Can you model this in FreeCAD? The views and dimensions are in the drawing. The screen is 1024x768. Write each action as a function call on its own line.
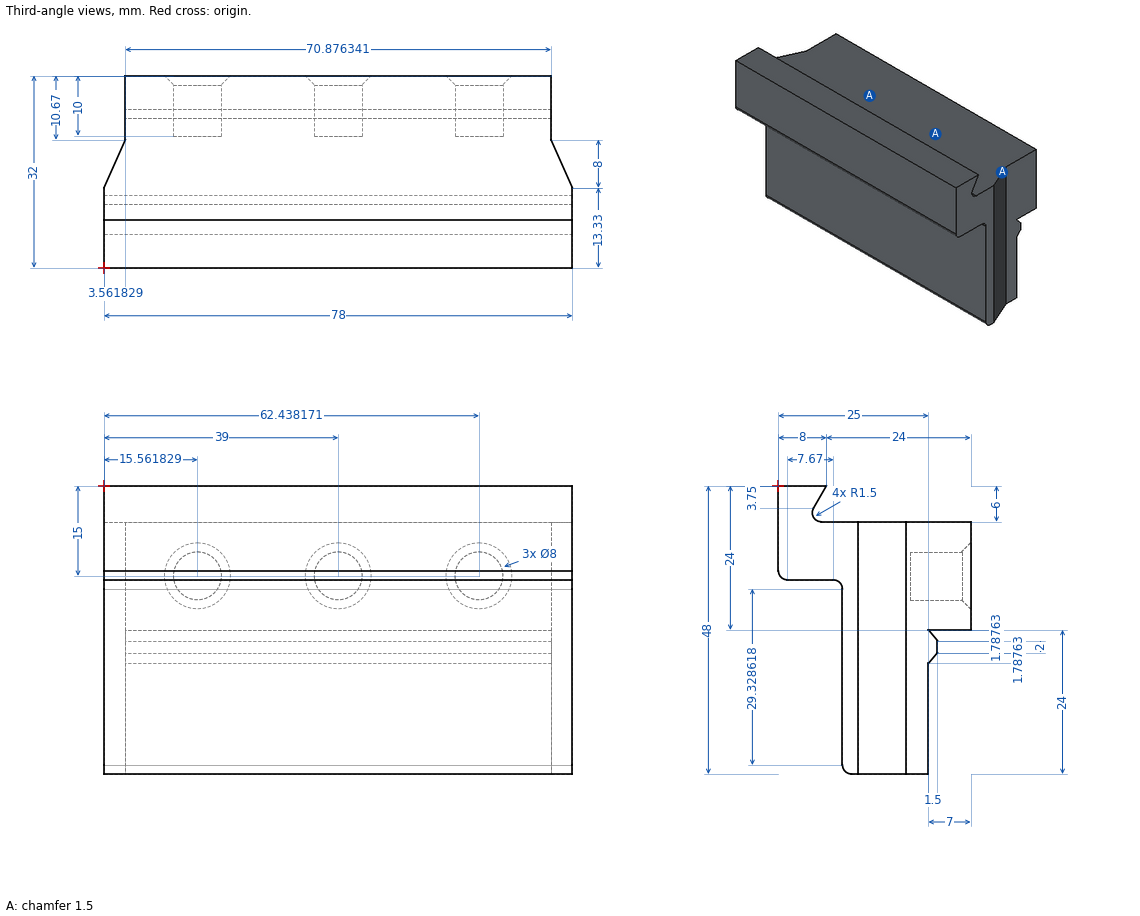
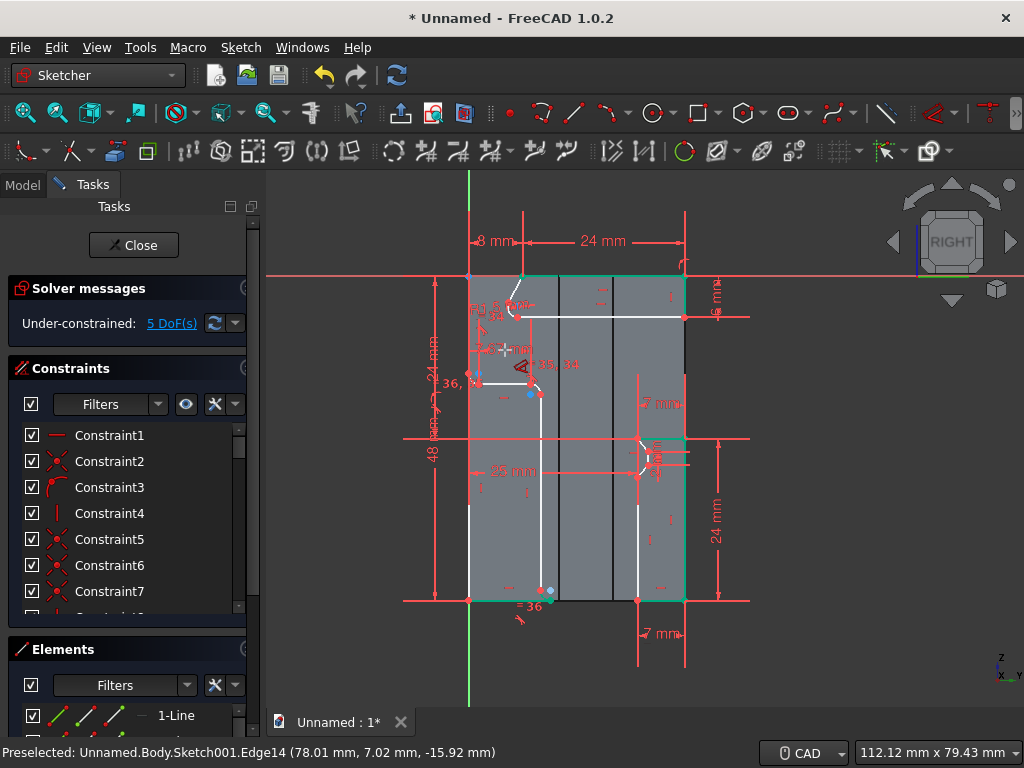
scroll(644, 447, up, 7)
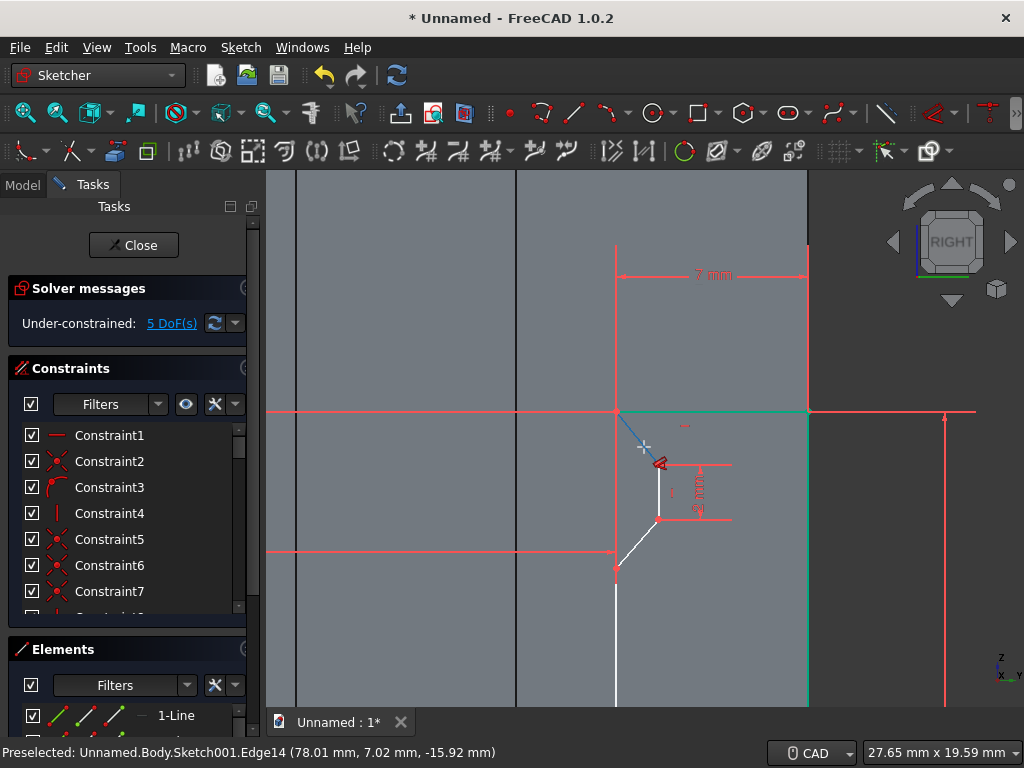
click(642, 444)
click(628, 499)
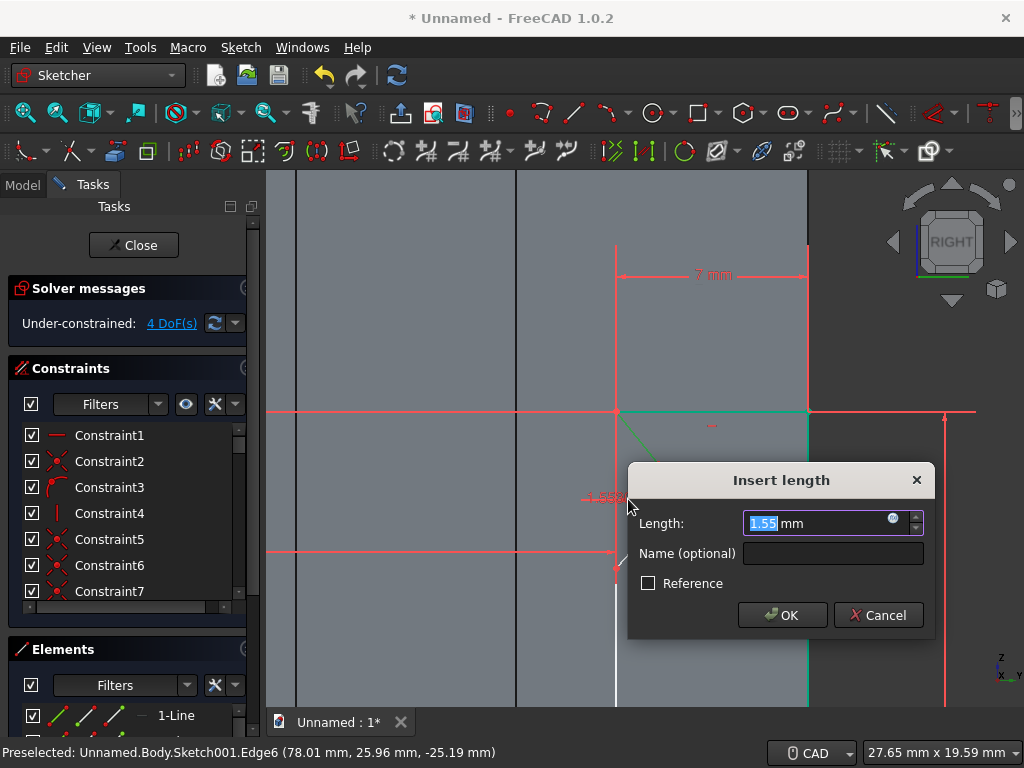
text(1.5)
key(Return)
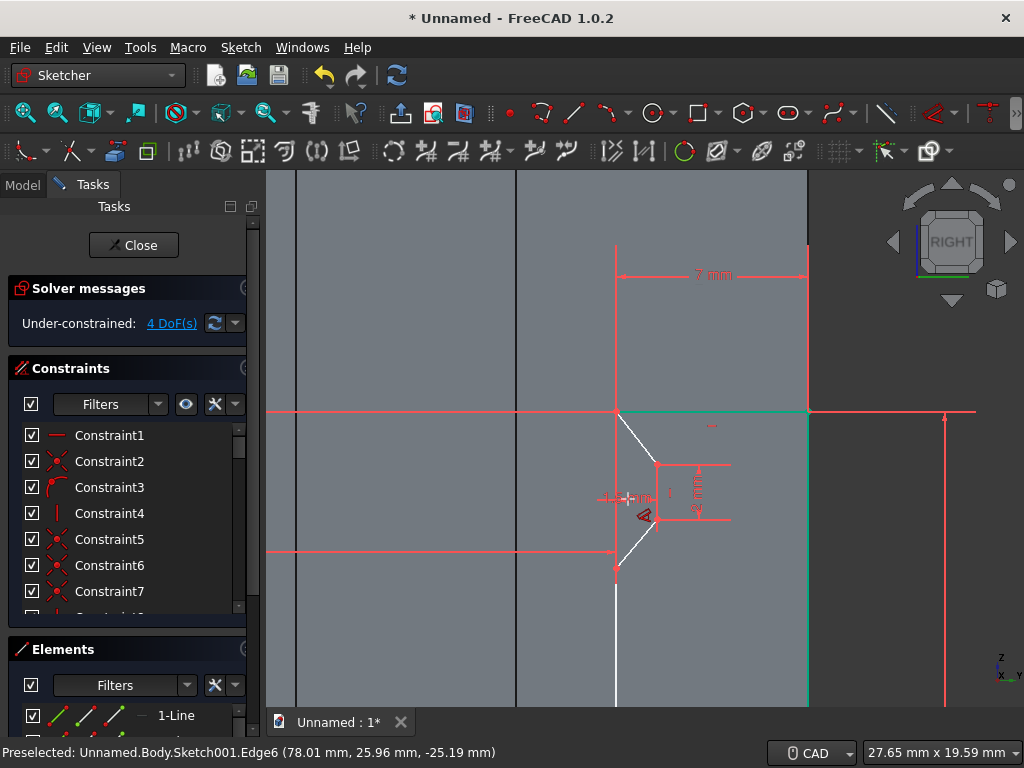
scroll(644, 447, down, 7)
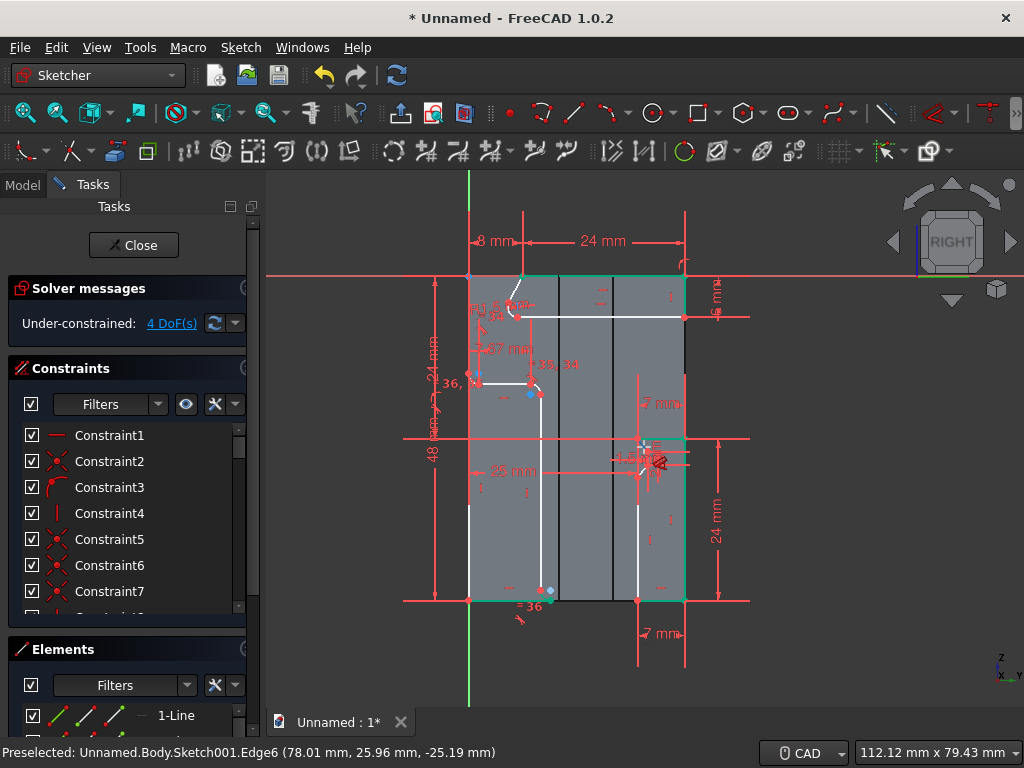
scroll(509, 302, up, 3)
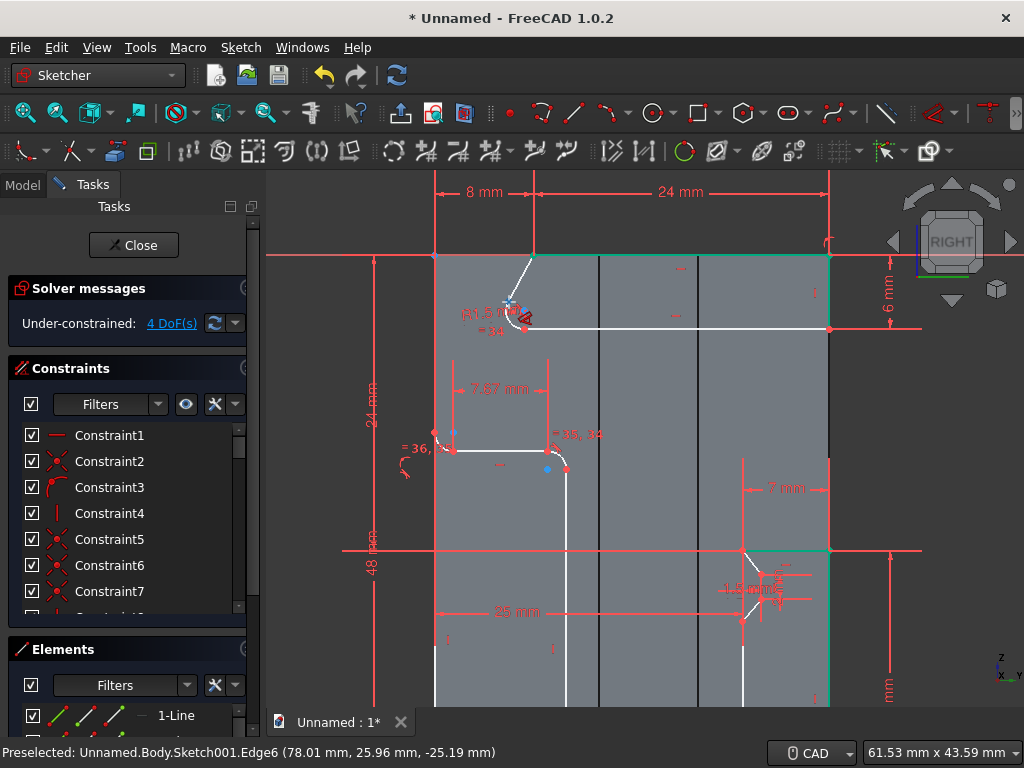
click(508, 302)
click(401, 279)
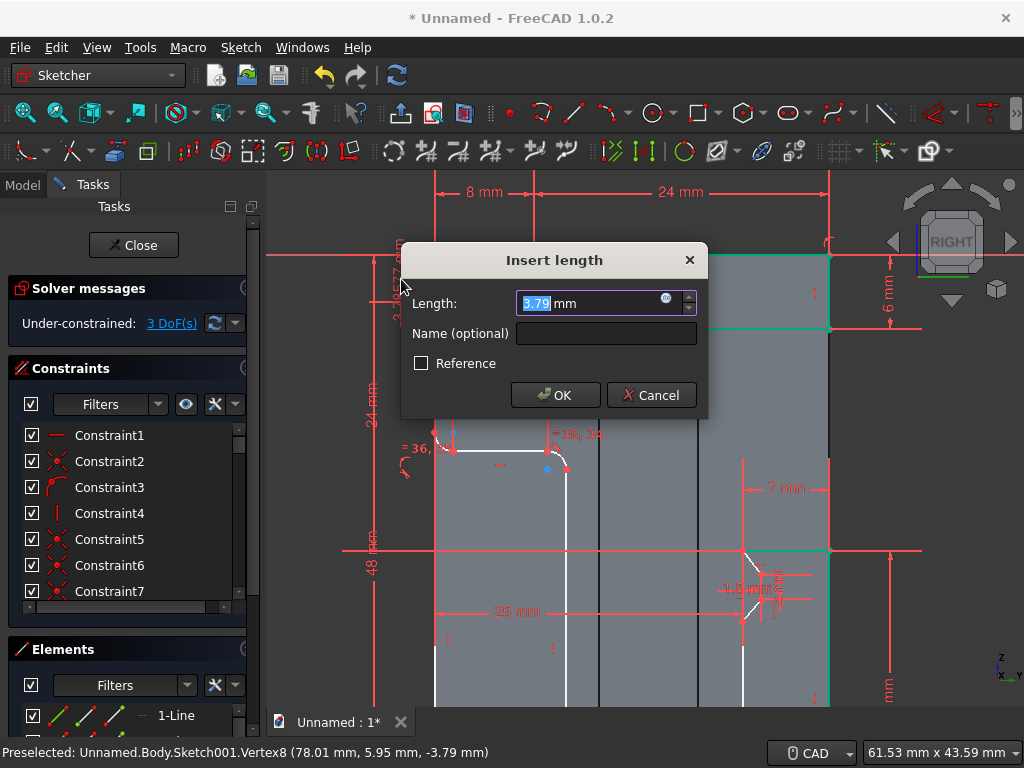
text(3.75)
key(Return)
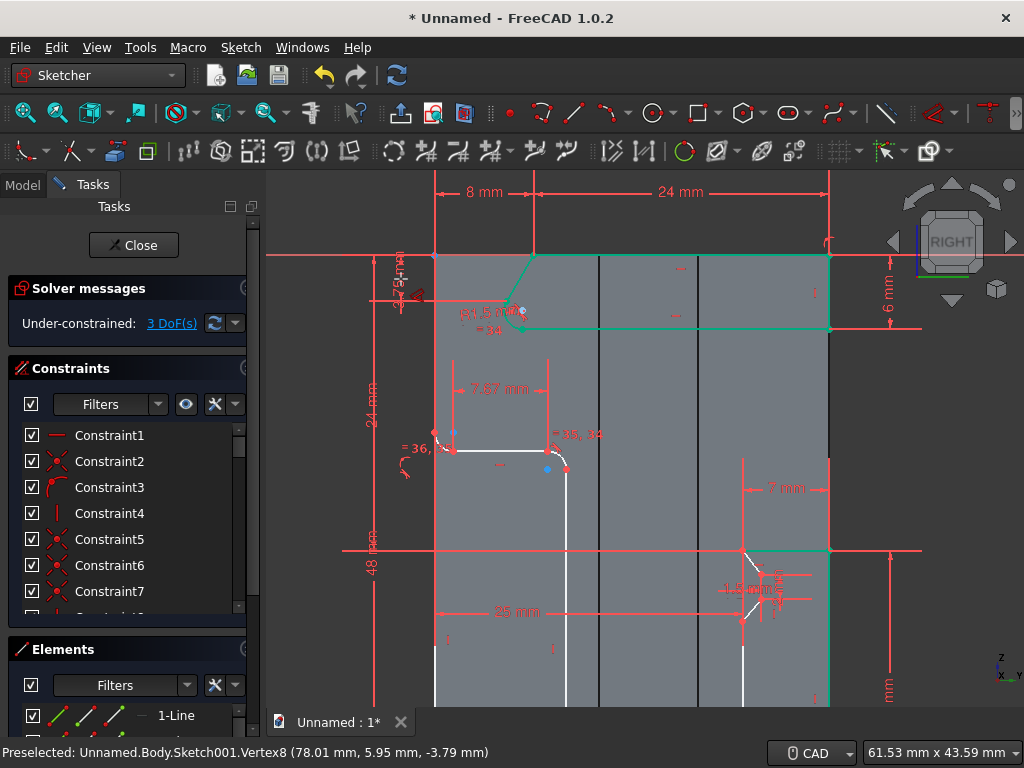
scroll(756, 568, up, 3)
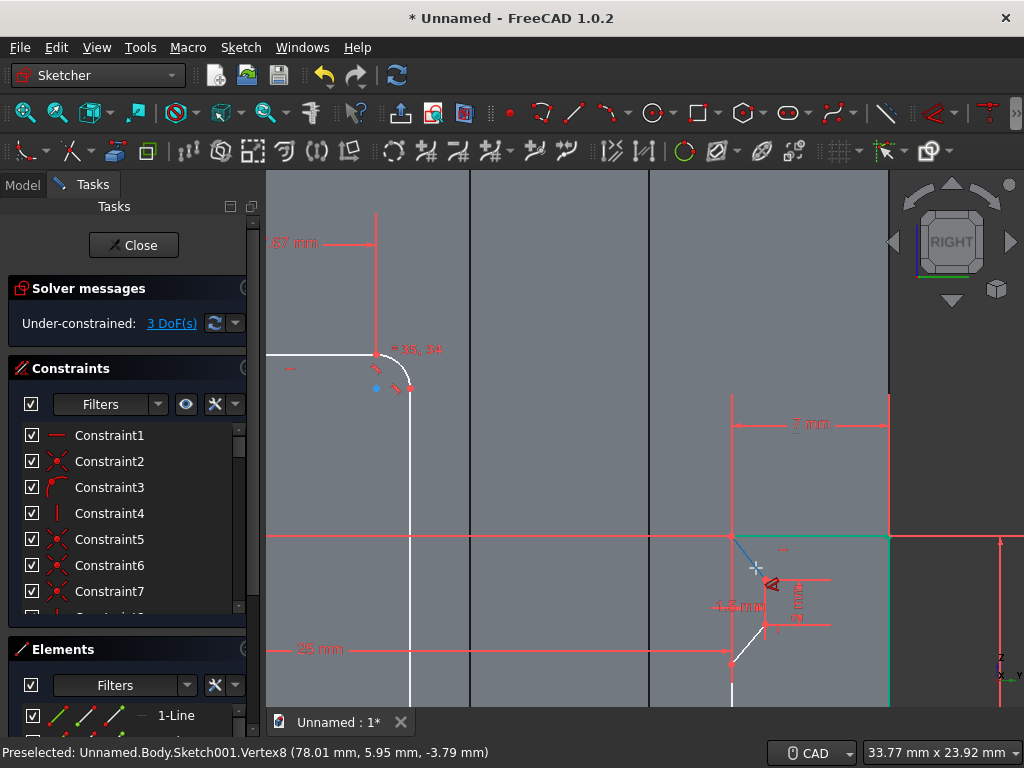
click(755, 567)
click(799, 558)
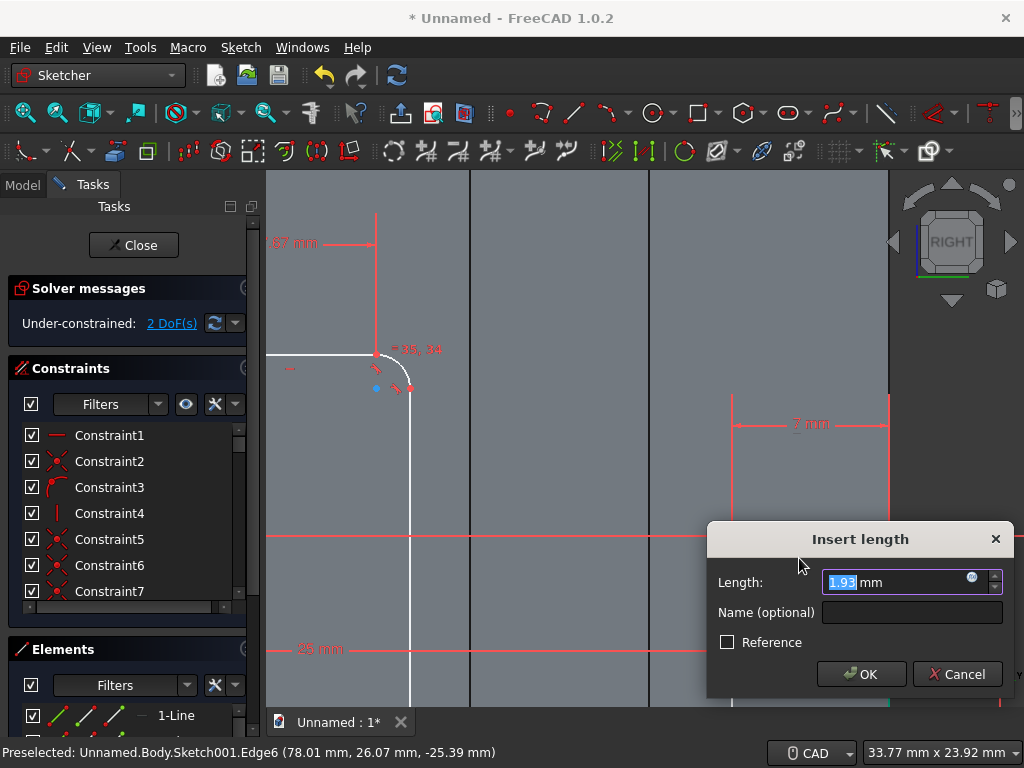
text(1.78763)
key(Return)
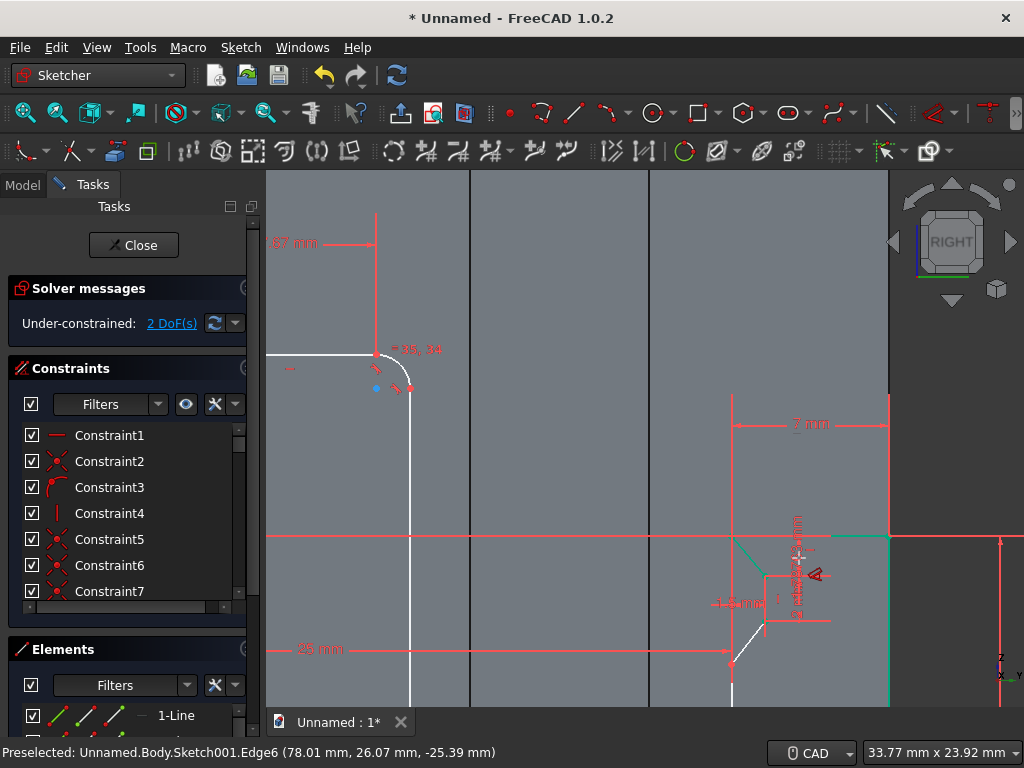
click(755, 634)
click(799, 643)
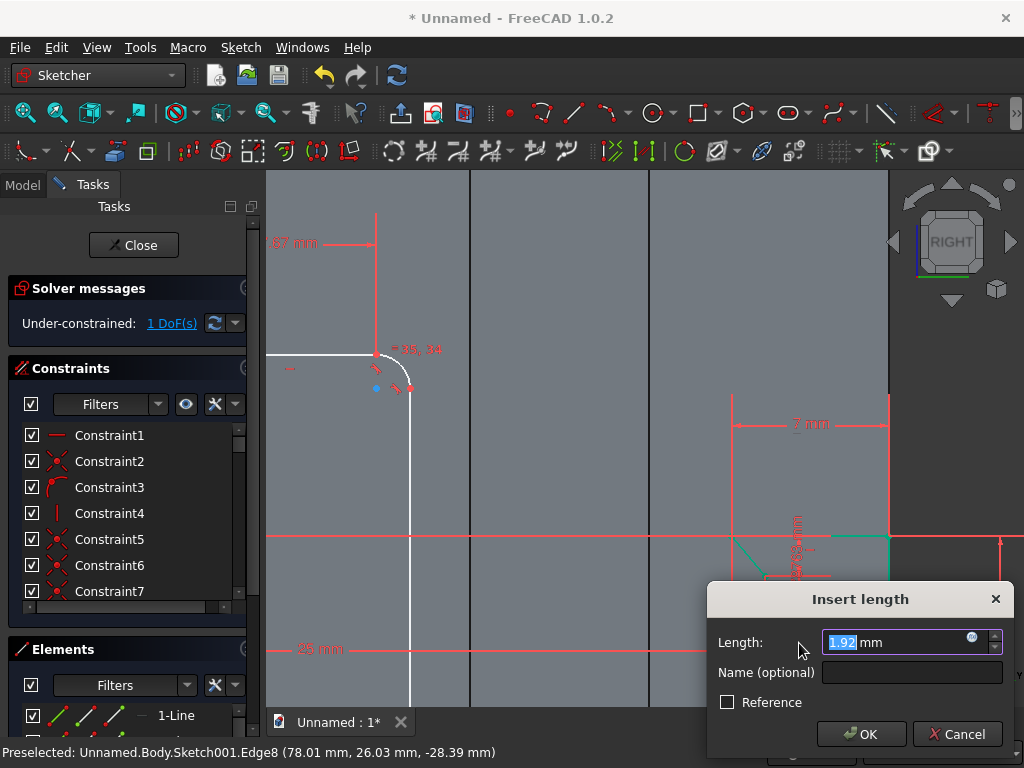
text(1.78763)
key(Return)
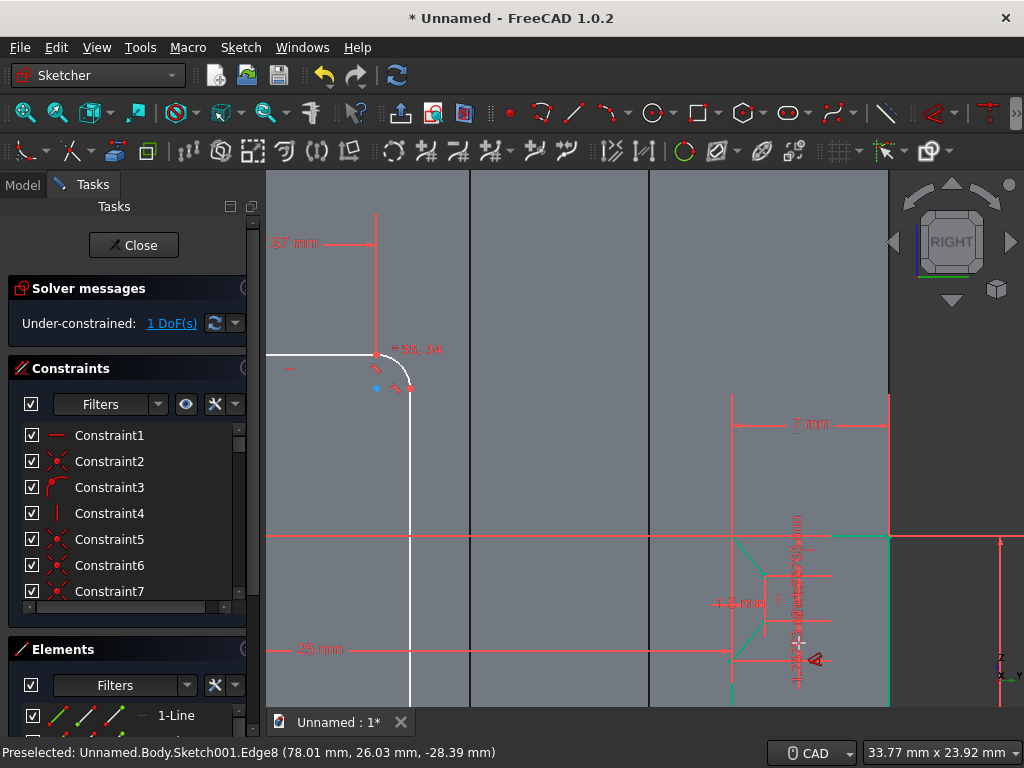
scroll(597, 396, down, 6)